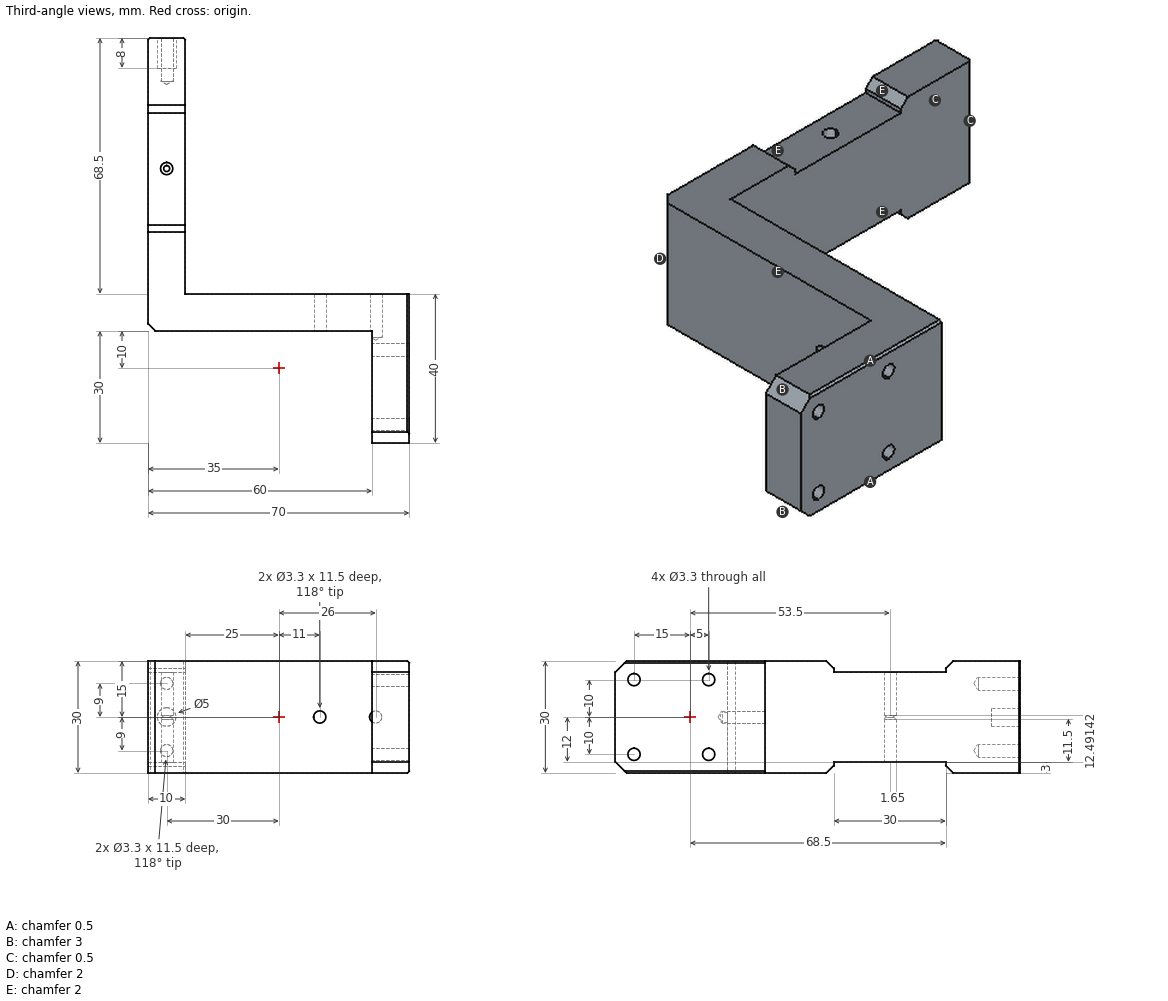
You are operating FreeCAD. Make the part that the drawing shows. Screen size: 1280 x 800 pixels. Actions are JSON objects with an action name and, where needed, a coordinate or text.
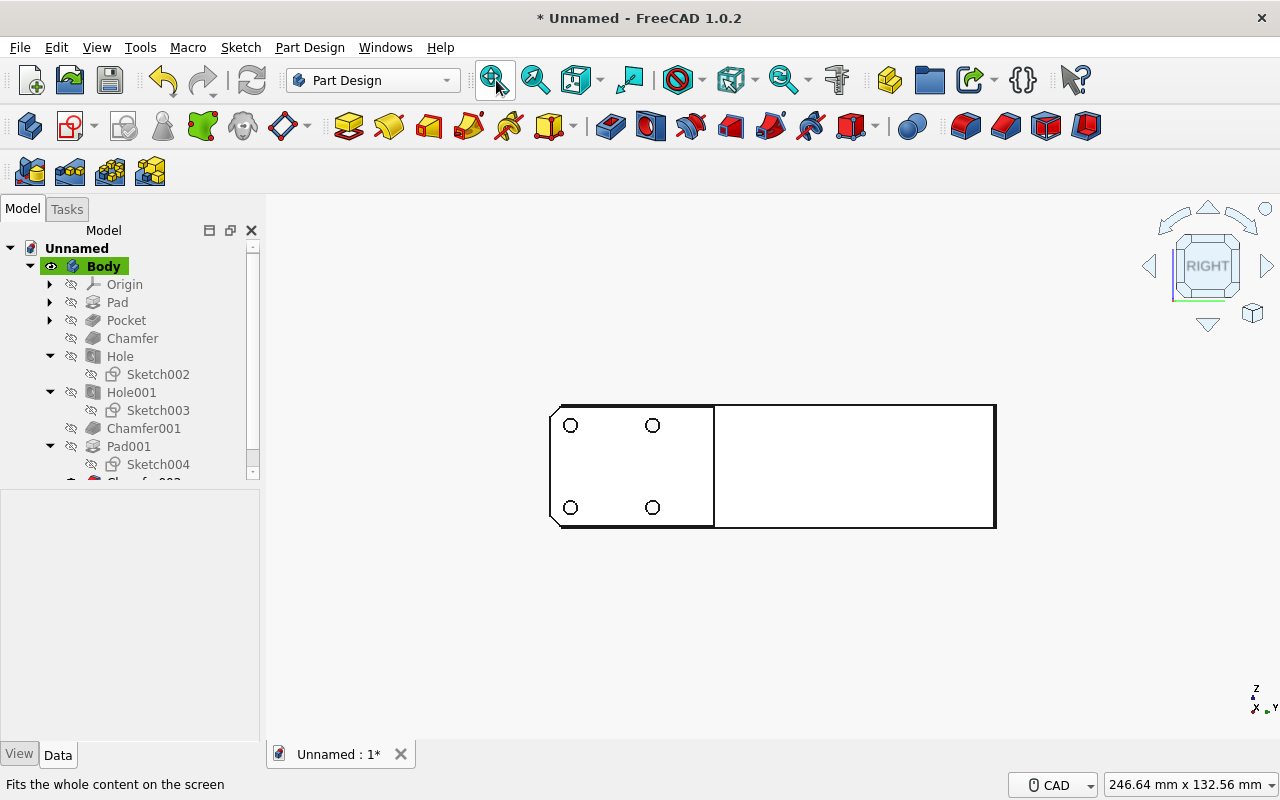
{"action": "key", "text": "4"}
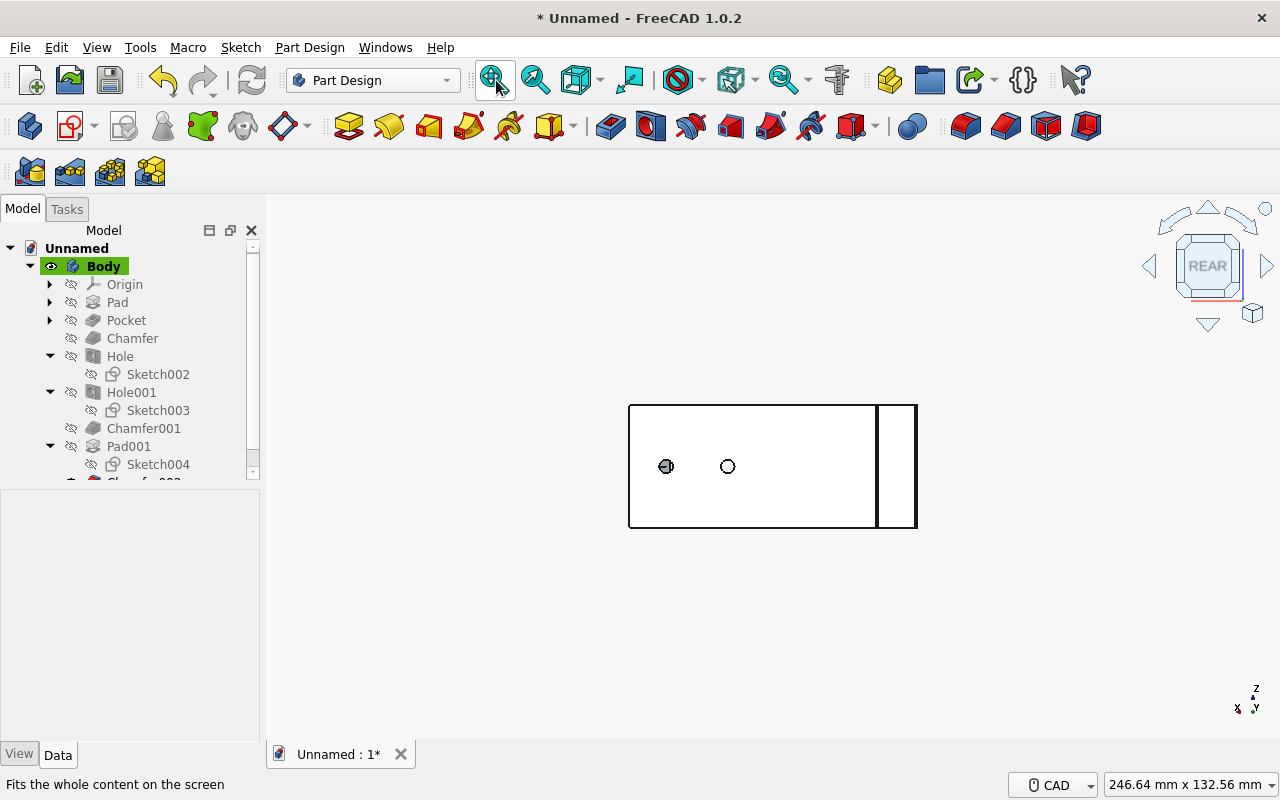
{"action": "left_click", "coordinate": [496, 80]}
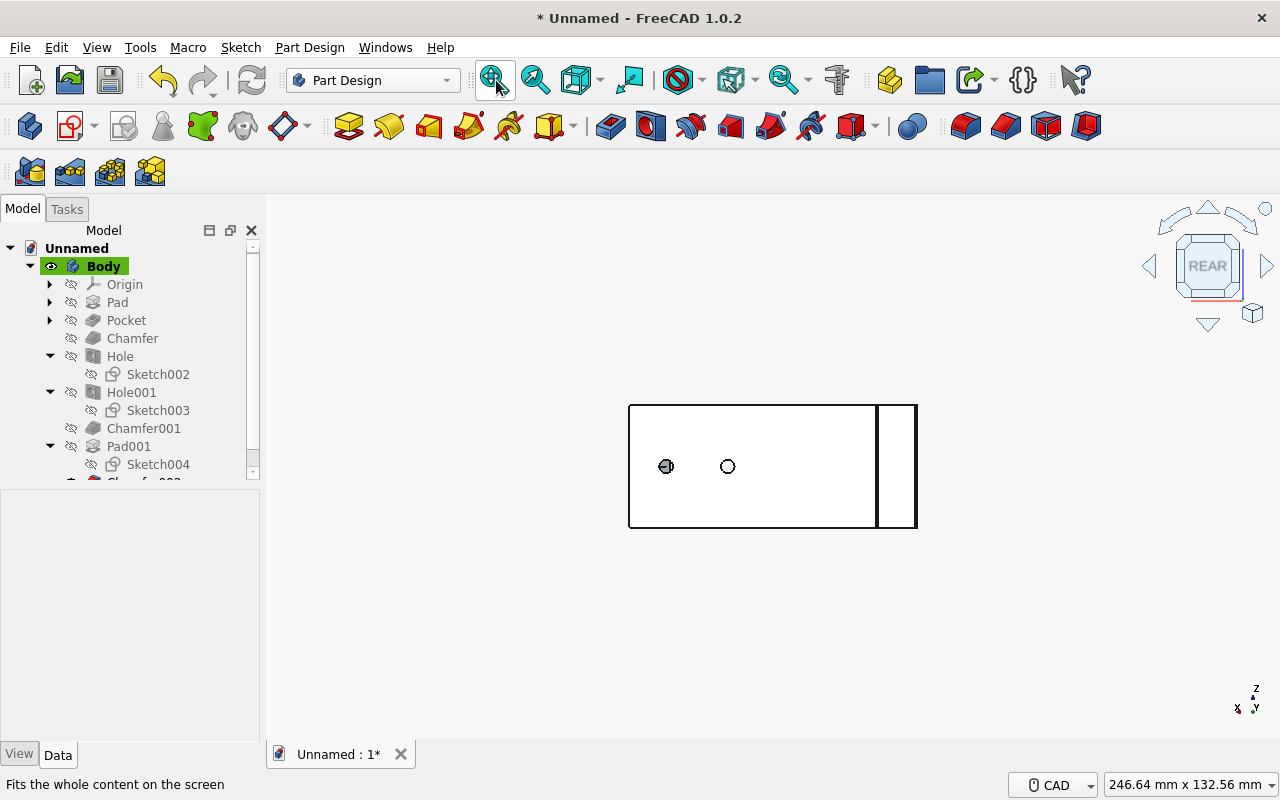
{"action": "left_click", "coordinate": [896, 430]}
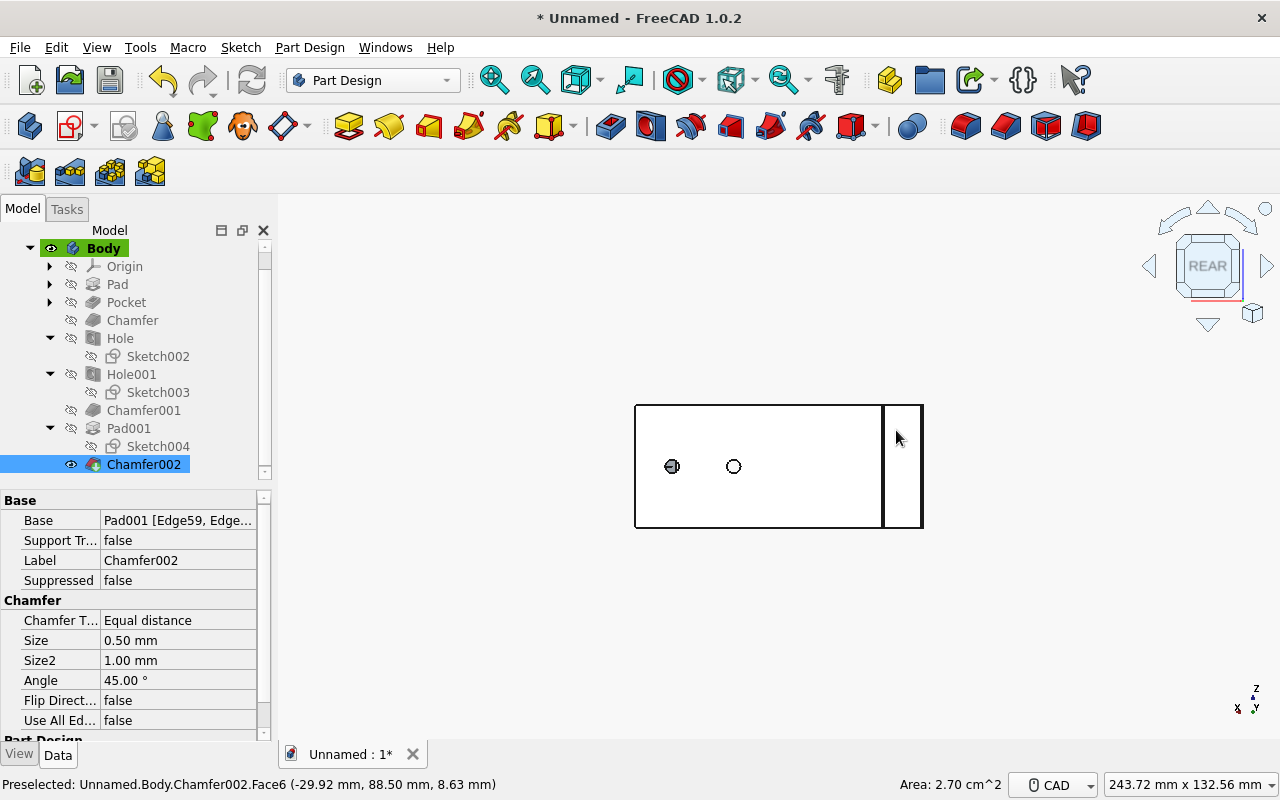
{"action": "left_click", "coordinate": [70, 126]}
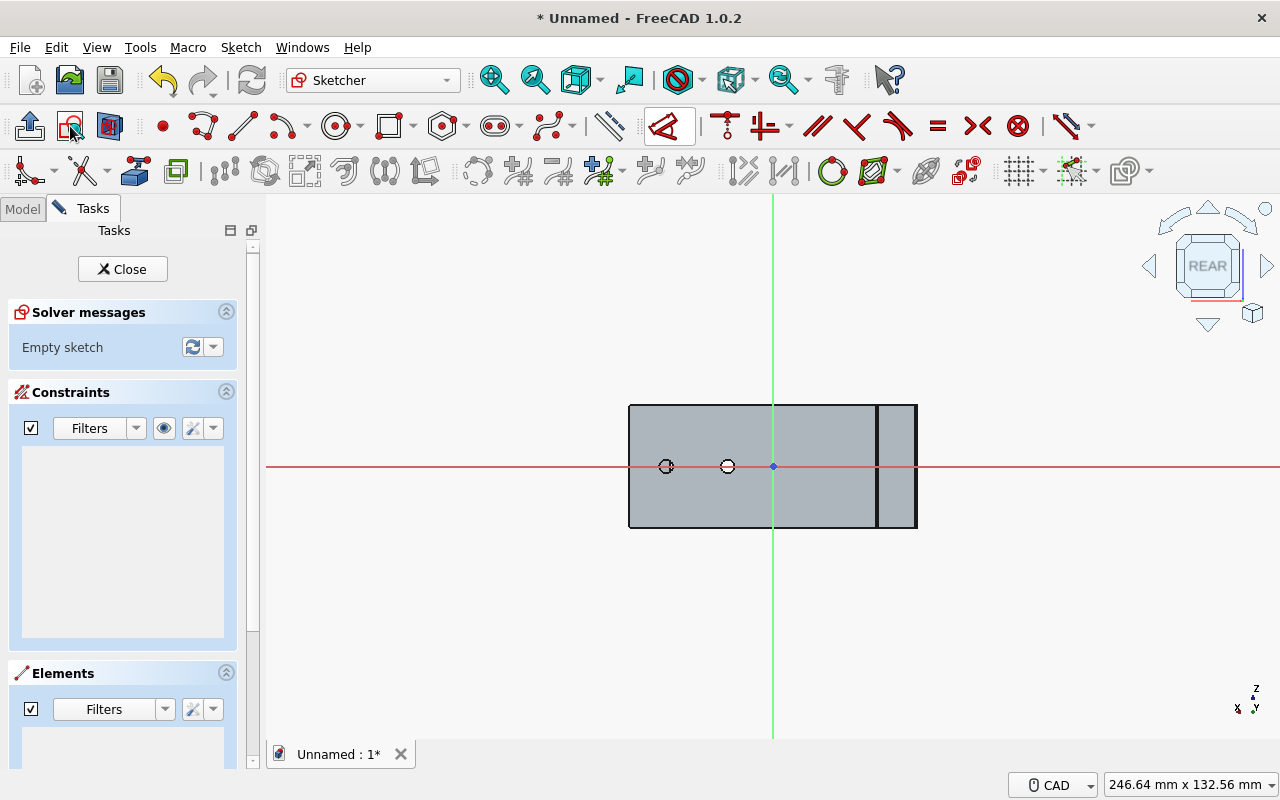
{"action": "scroll", "coordinate": [882, 467], "scroll_direction": "up", "scroll_amount": 7}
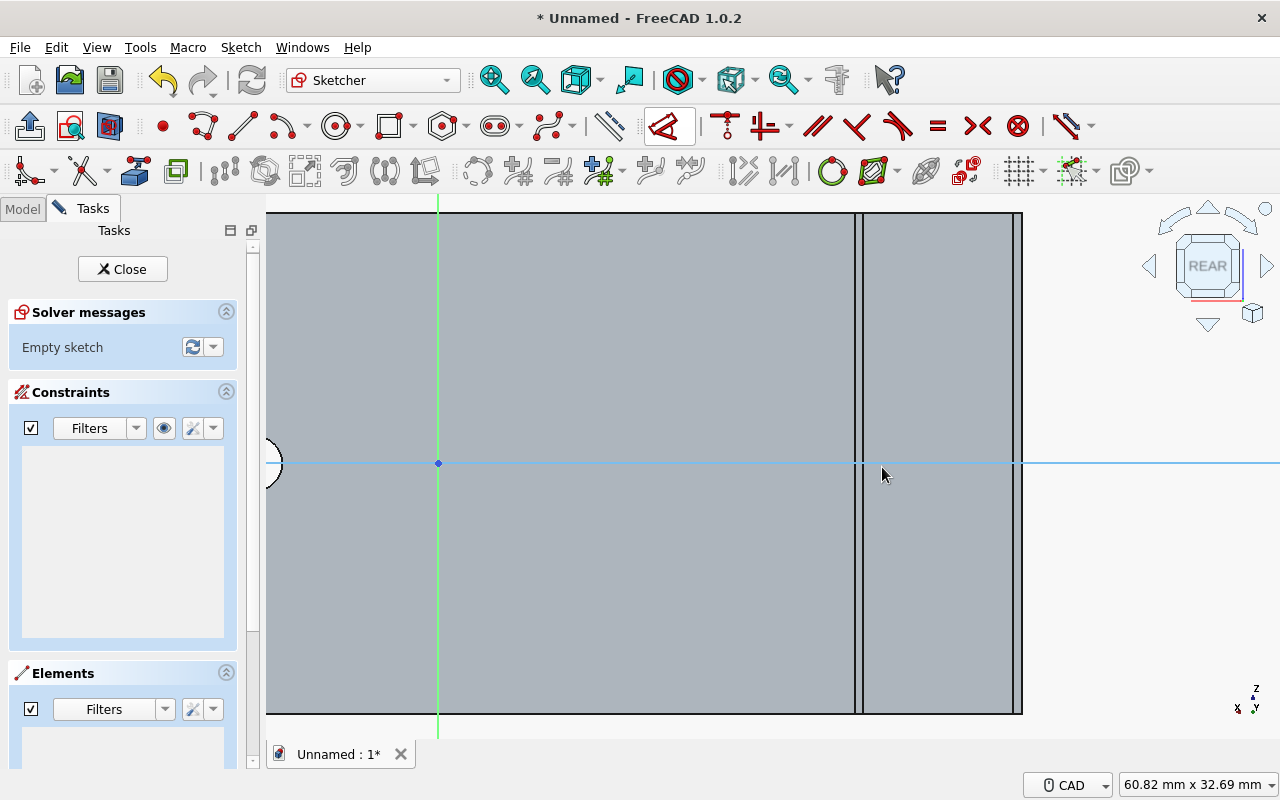
{"action": "left_click", "coordinate": [336, 126]}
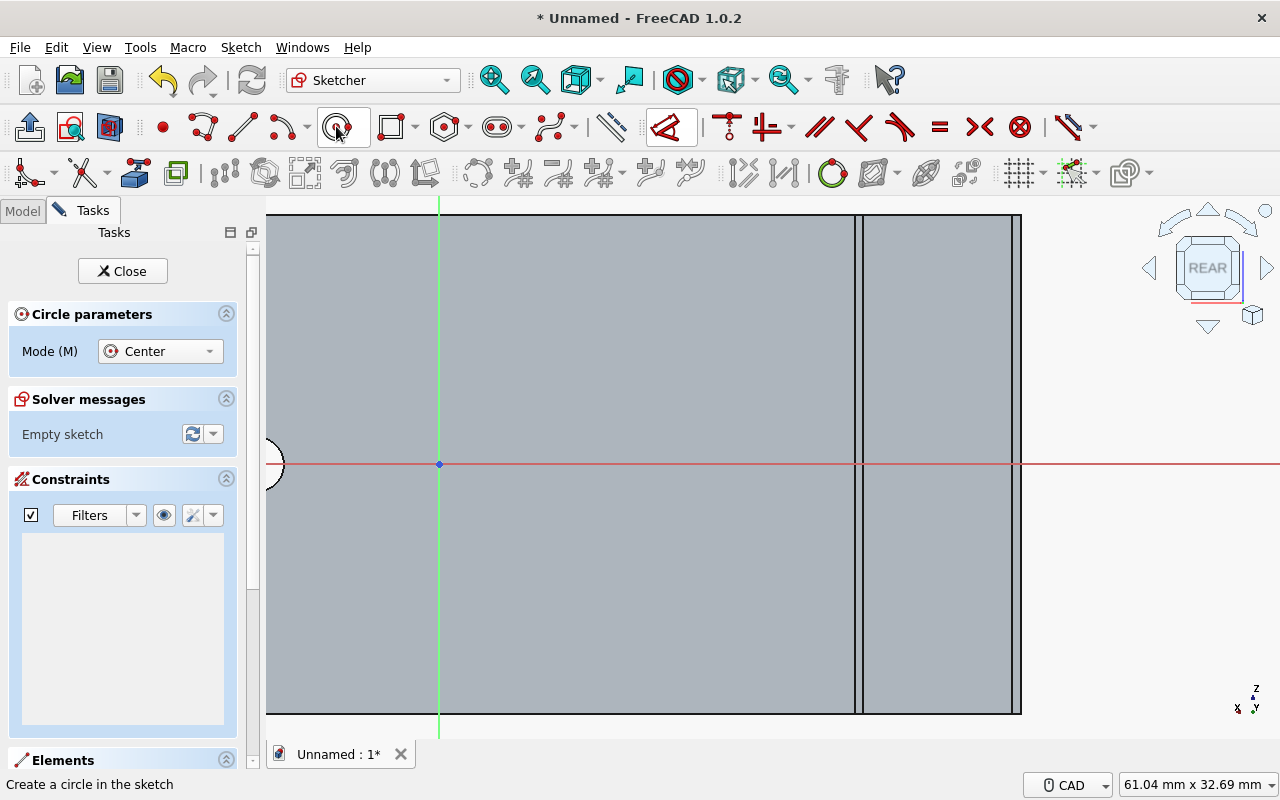
{"action": "left_click", "coordinate": [938, 614]}
{"action": "left_click", "coordinate": [957, 595]}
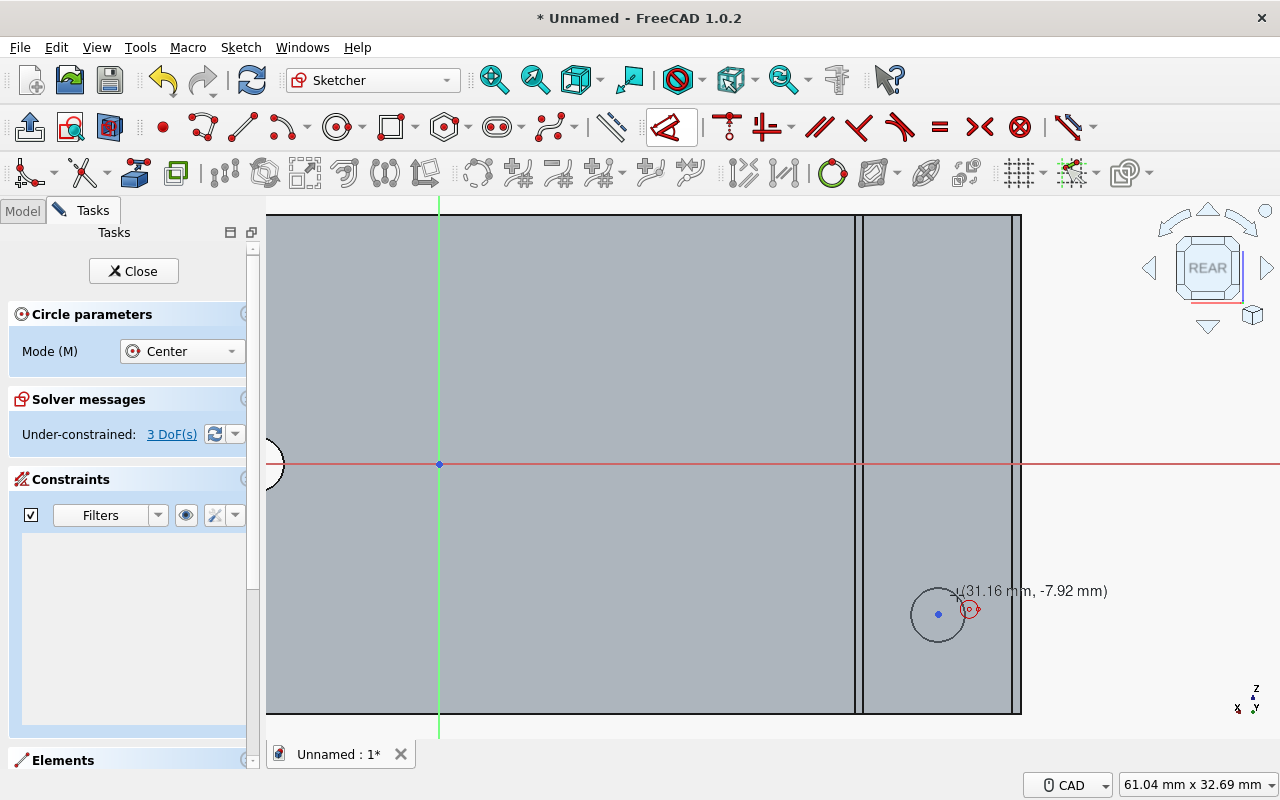
{"action": "left_click", "coordinate": [938, 315]}
{"action": "left_click", "coordinate": [957, 296]}
{"action": "key", "text": "Escape"}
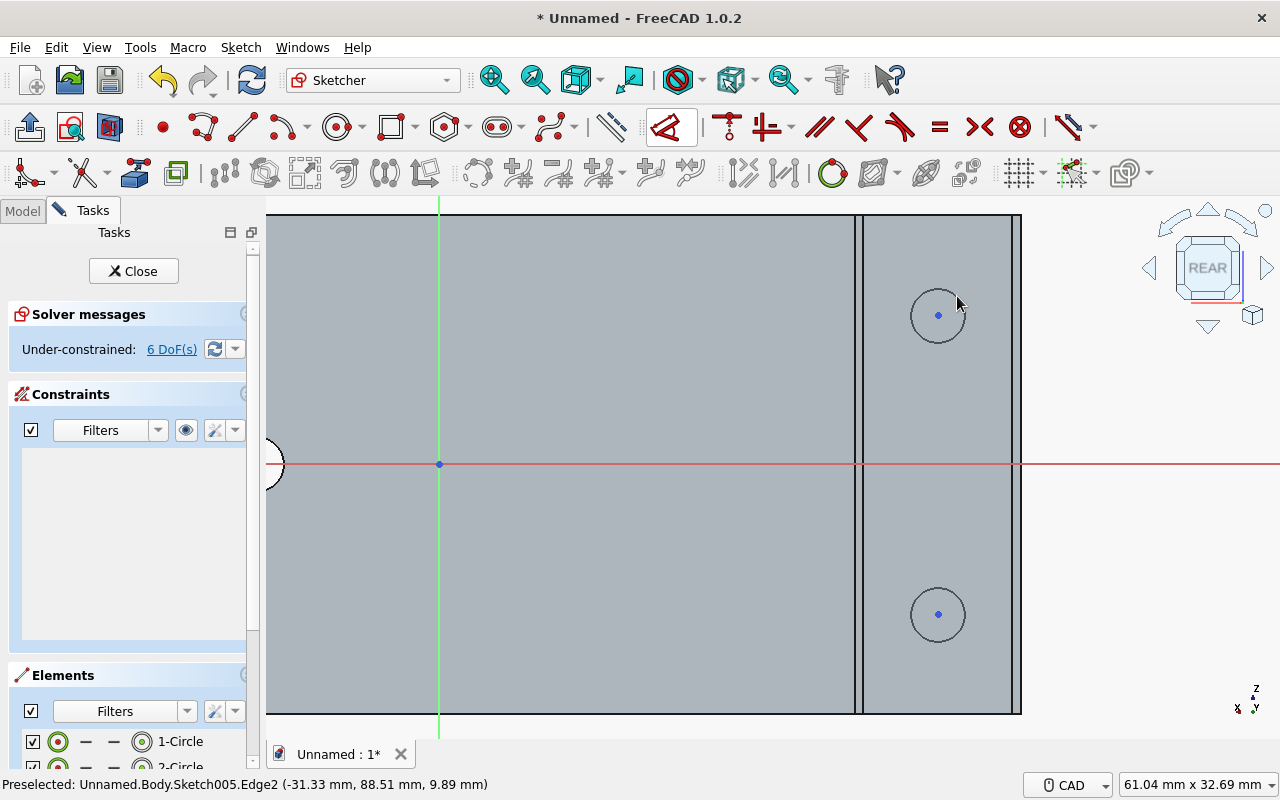
{"action": "left_click", "coordinate": [957, 596]}